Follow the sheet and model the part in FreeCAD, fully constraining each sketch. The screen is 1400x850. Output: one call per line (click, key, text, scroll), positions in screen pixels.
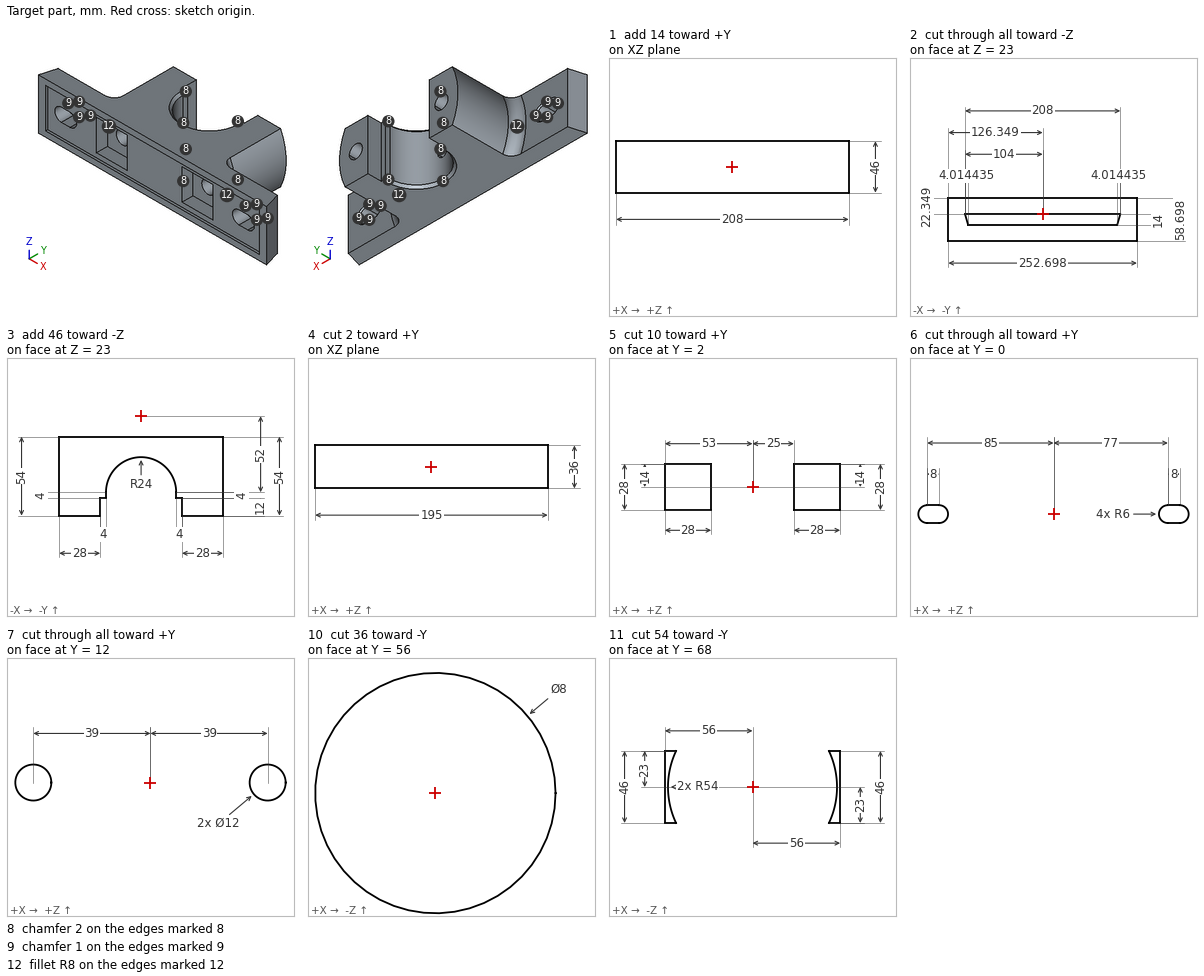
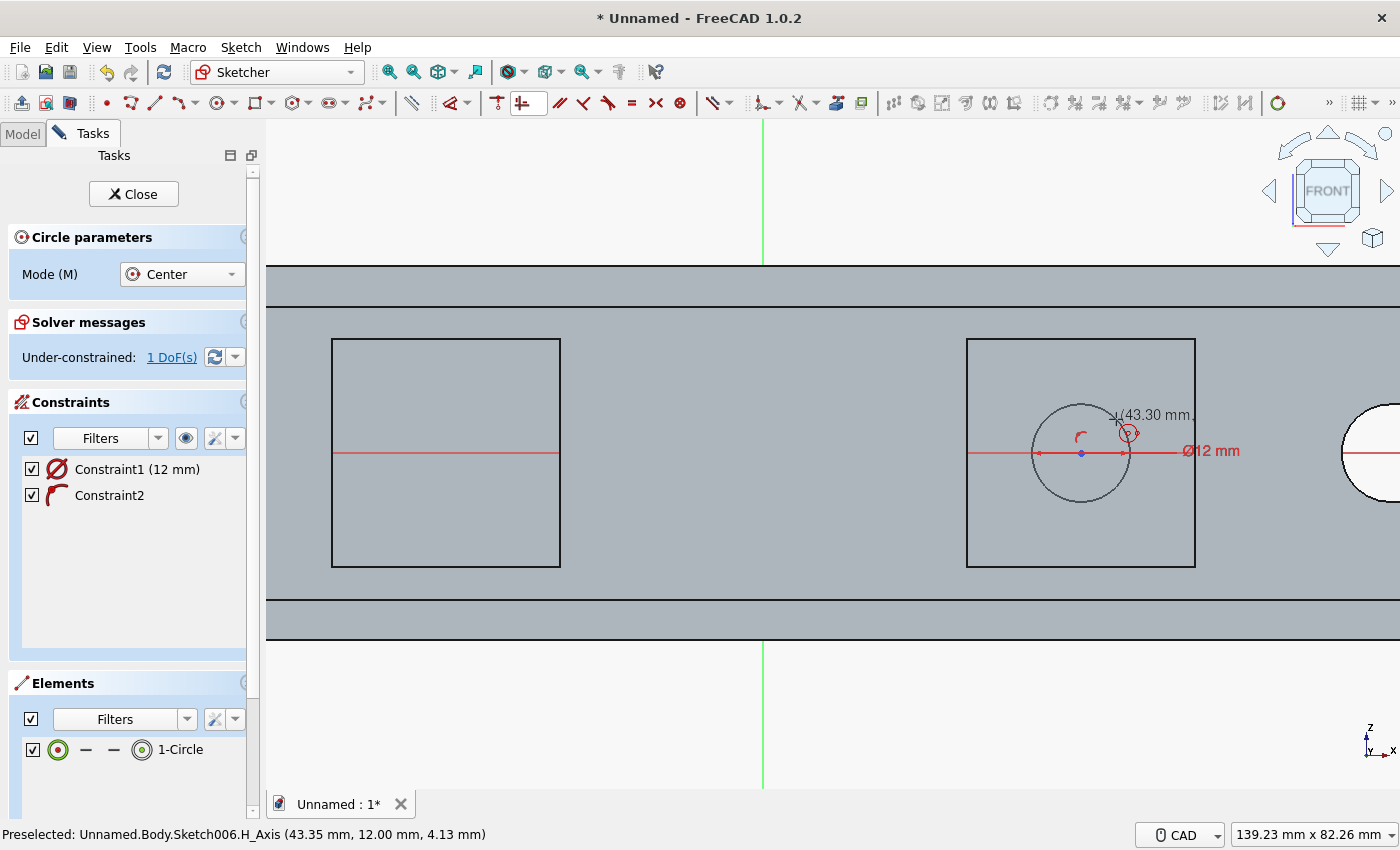
click(446, 453)
move(480, 419)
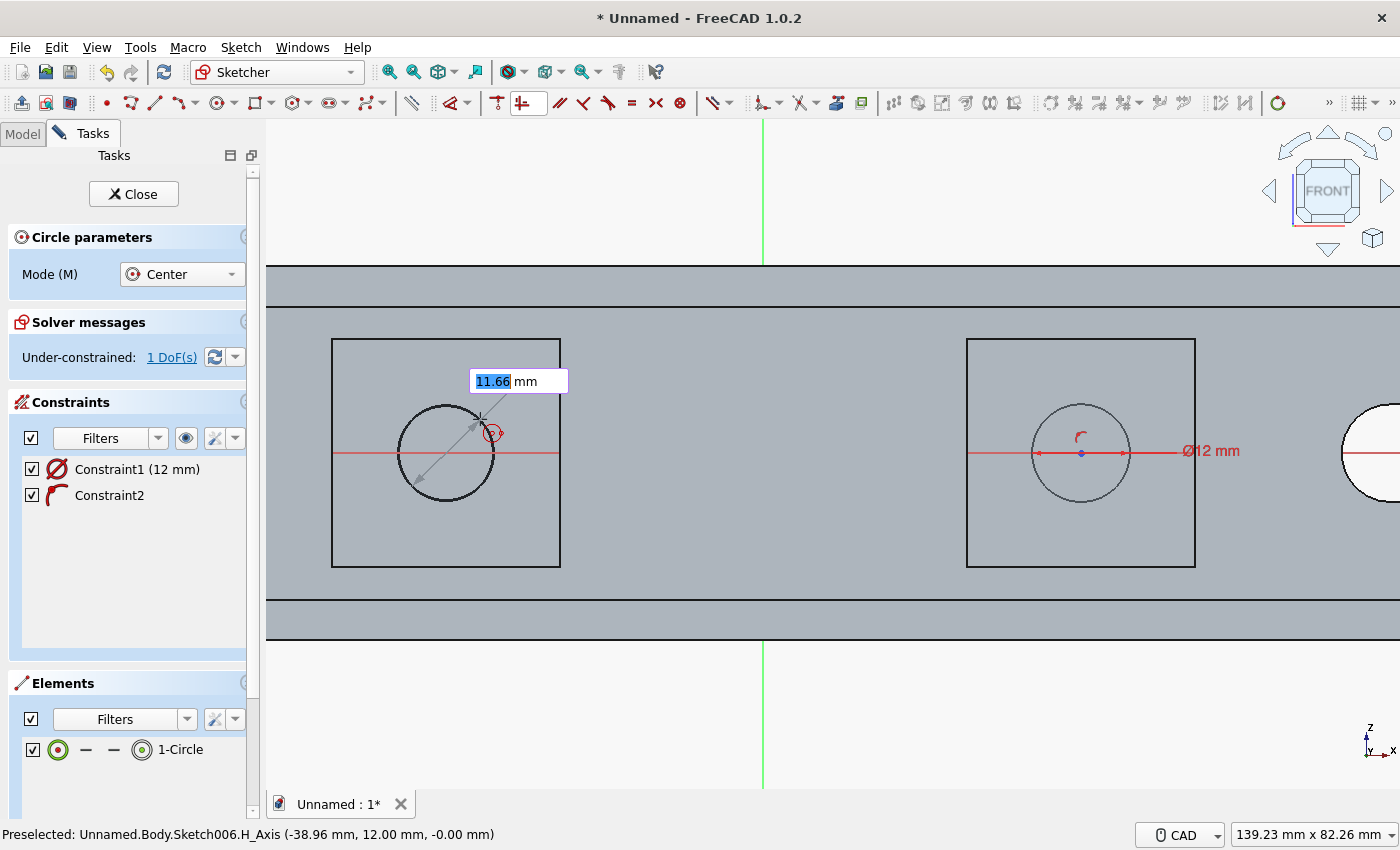
text(12)
key(Return)
key(Escape)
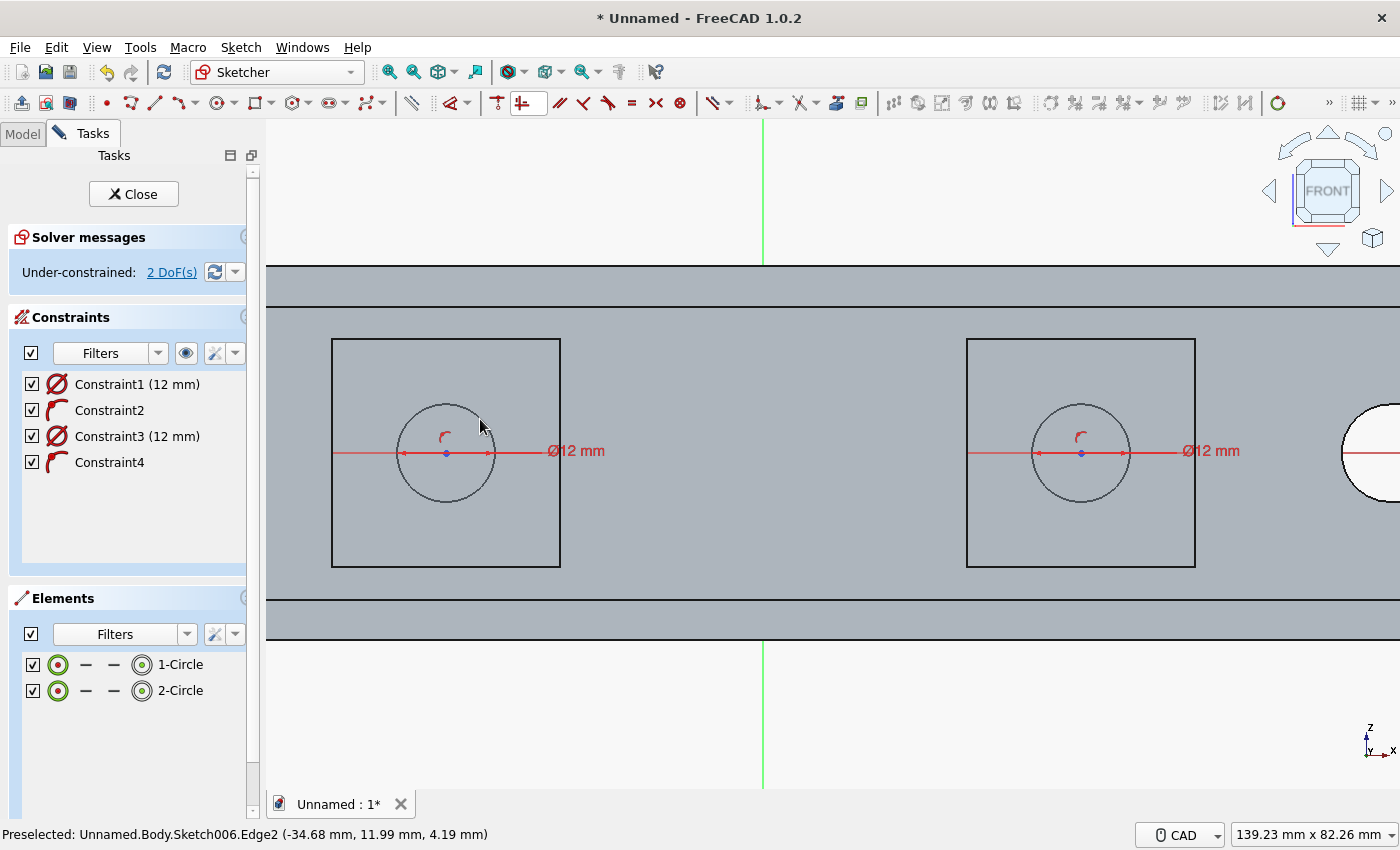
key(d)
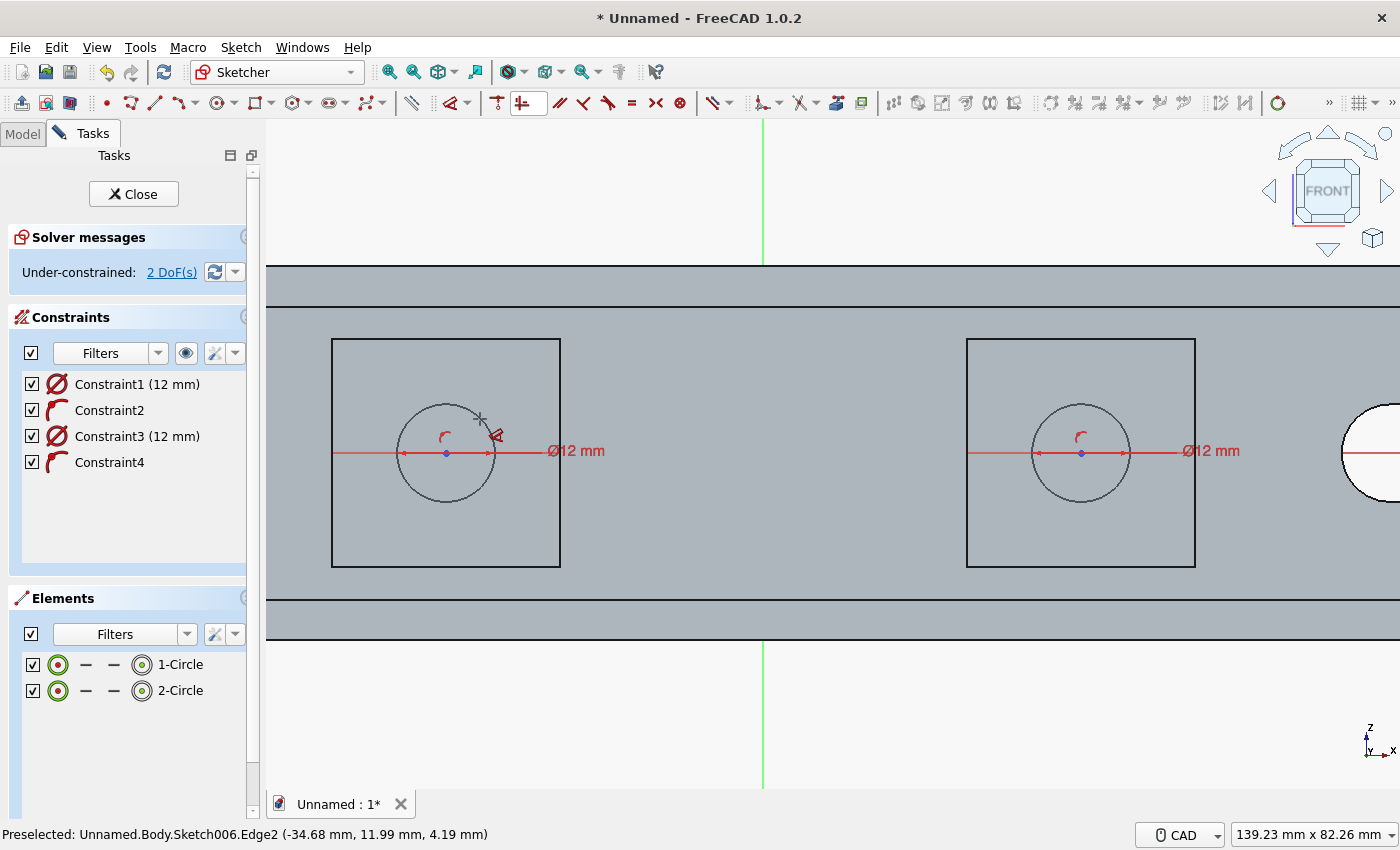
click(1081, 453)
click(922, 487)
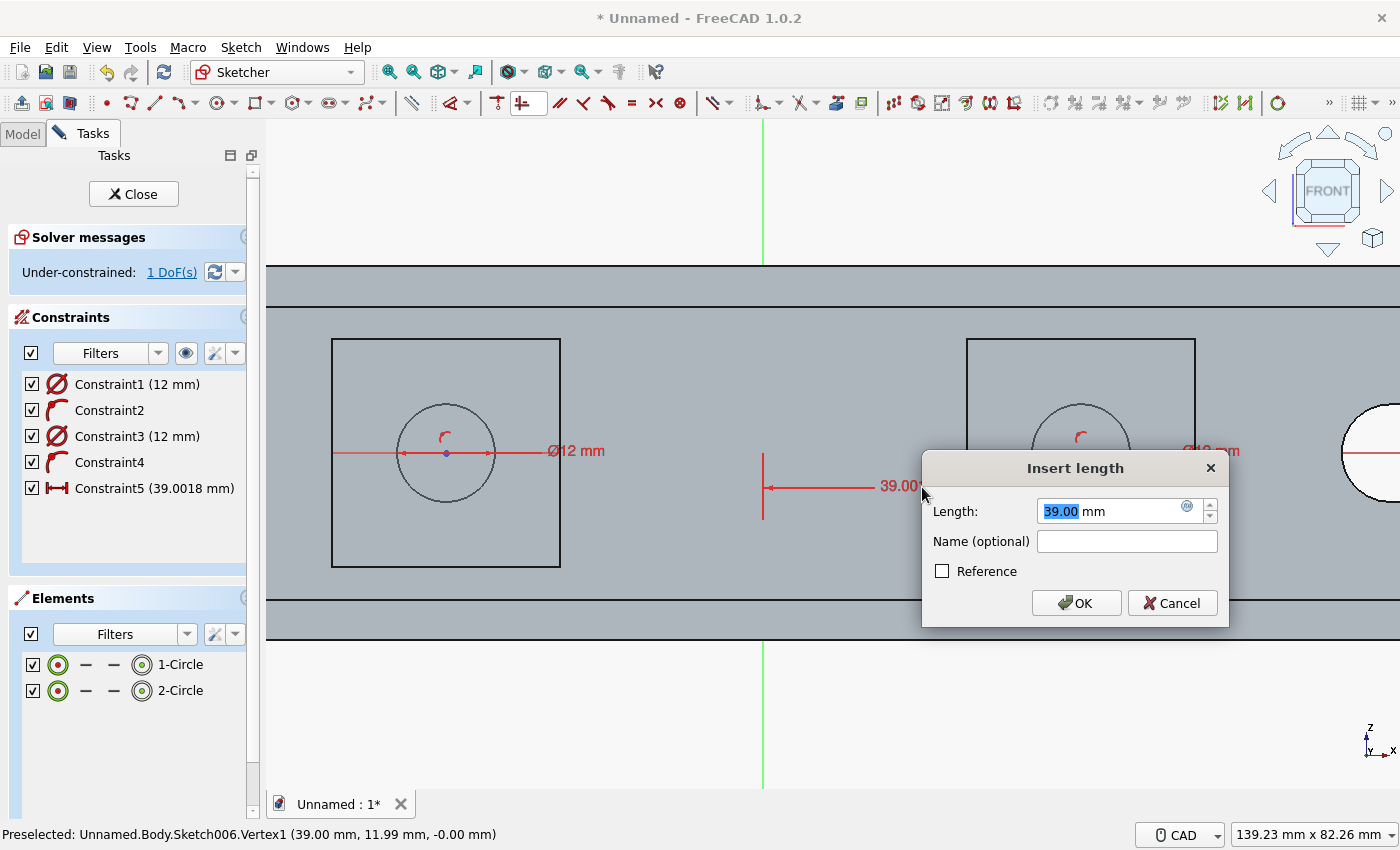
text(39)
key(Return)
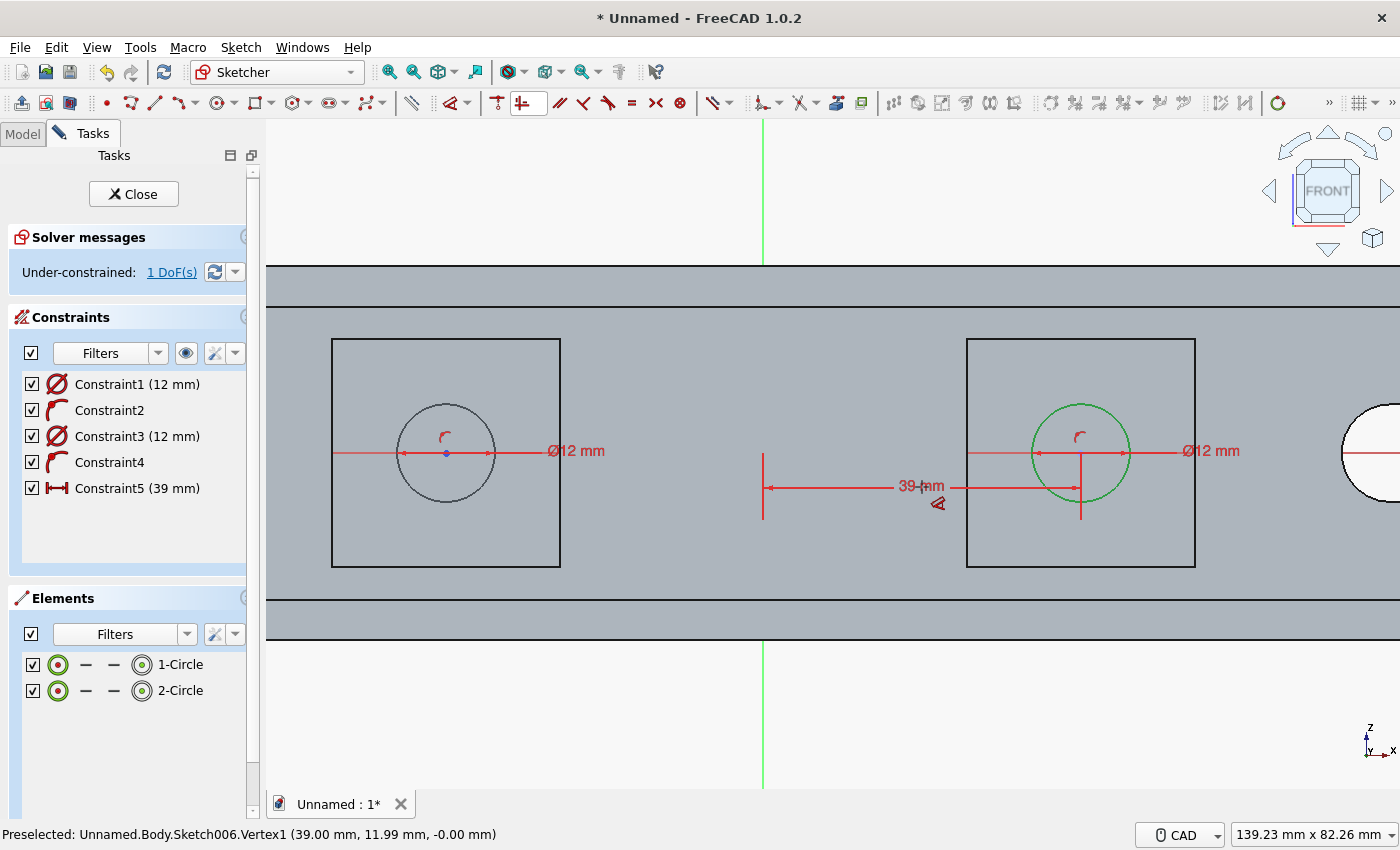
click(446, 453)
click(605, 487)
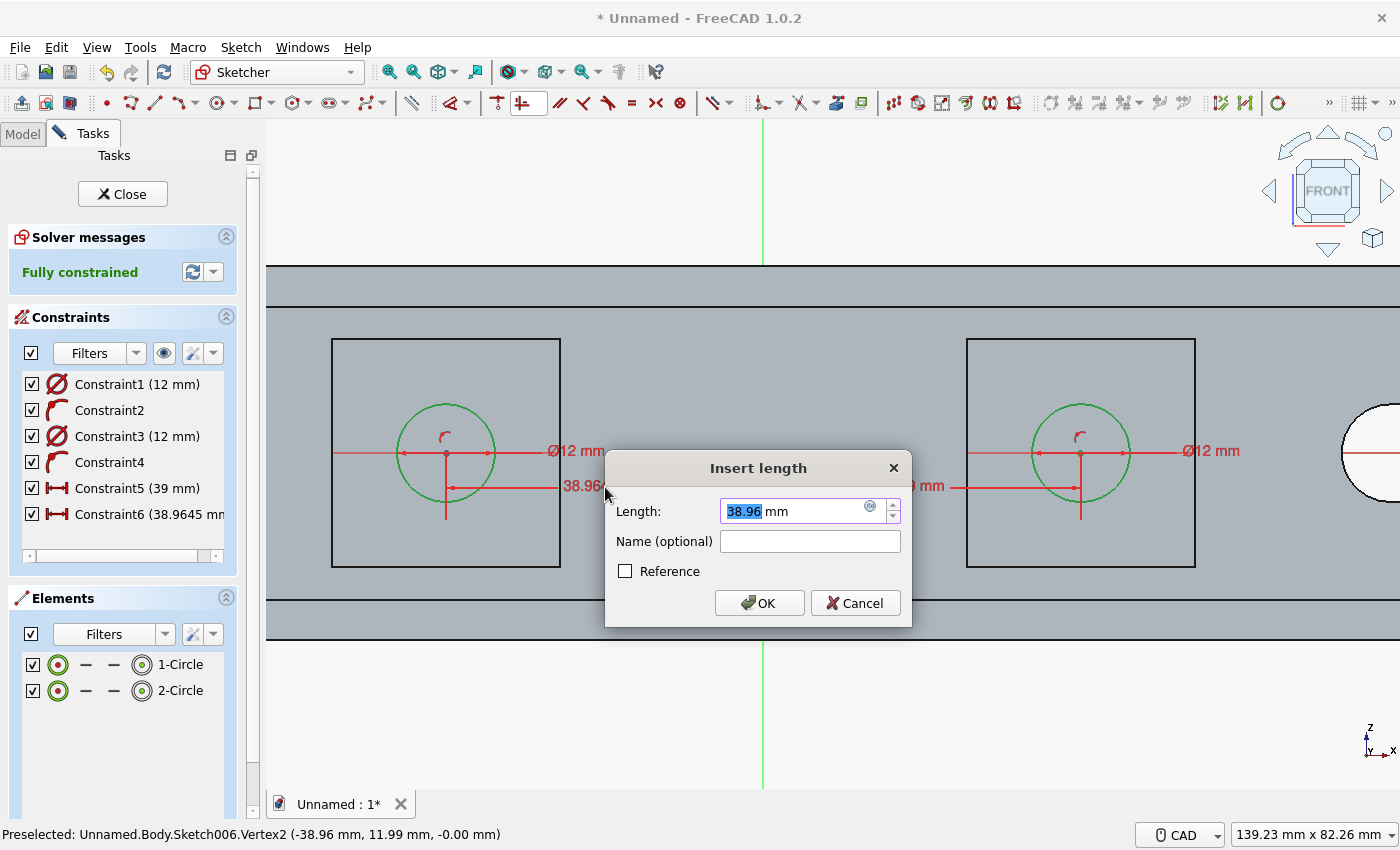
text(39)
key(Return)
key(Escape)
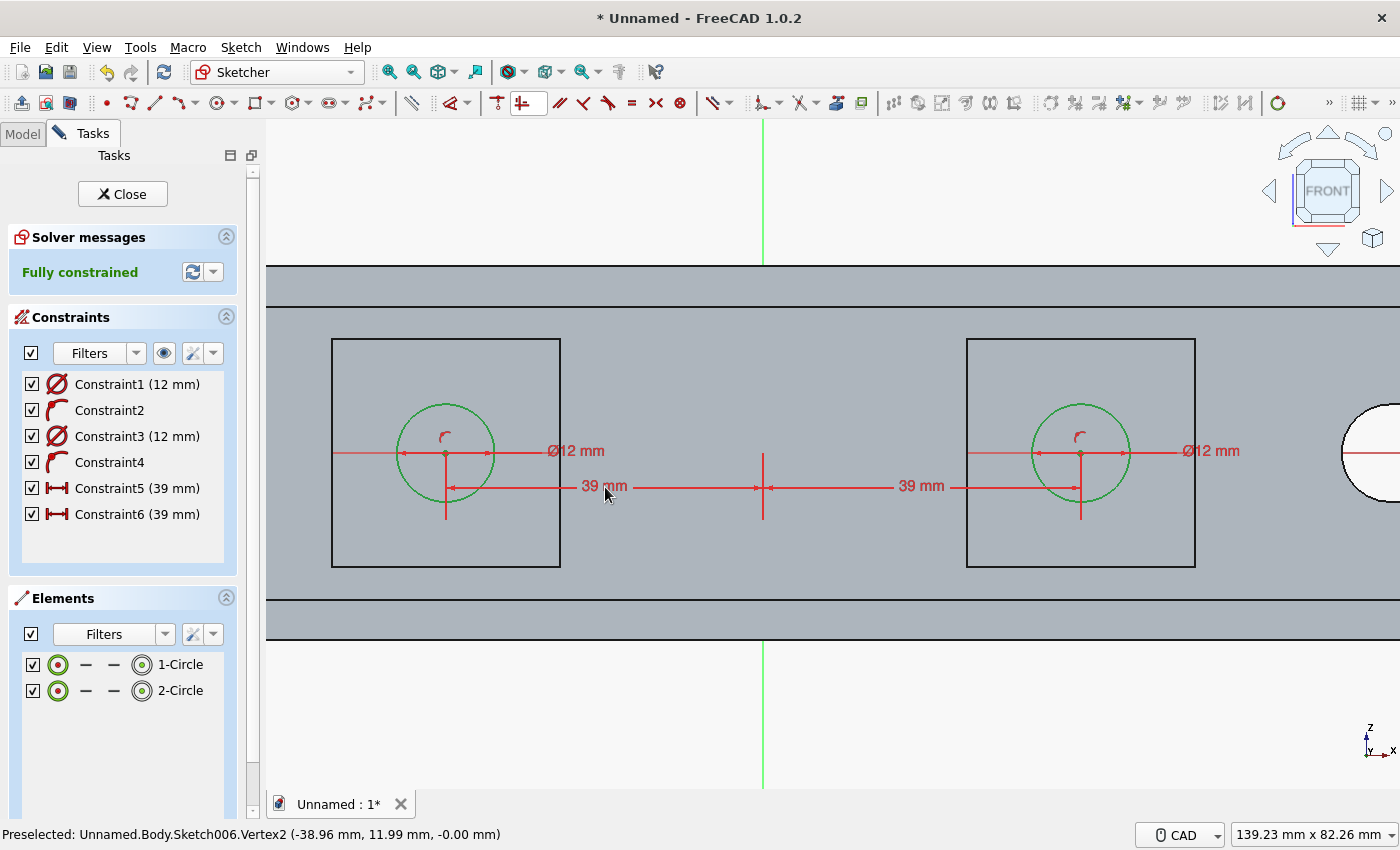
click(123, 194)